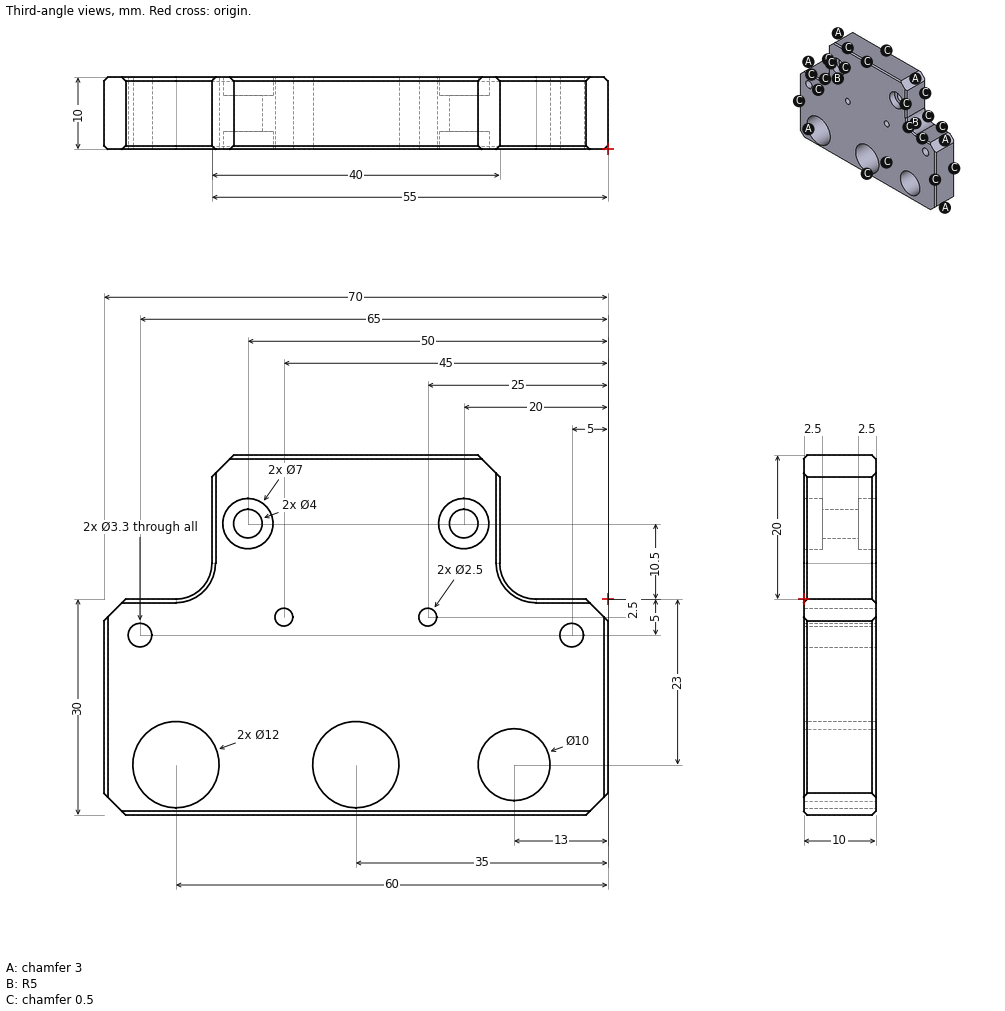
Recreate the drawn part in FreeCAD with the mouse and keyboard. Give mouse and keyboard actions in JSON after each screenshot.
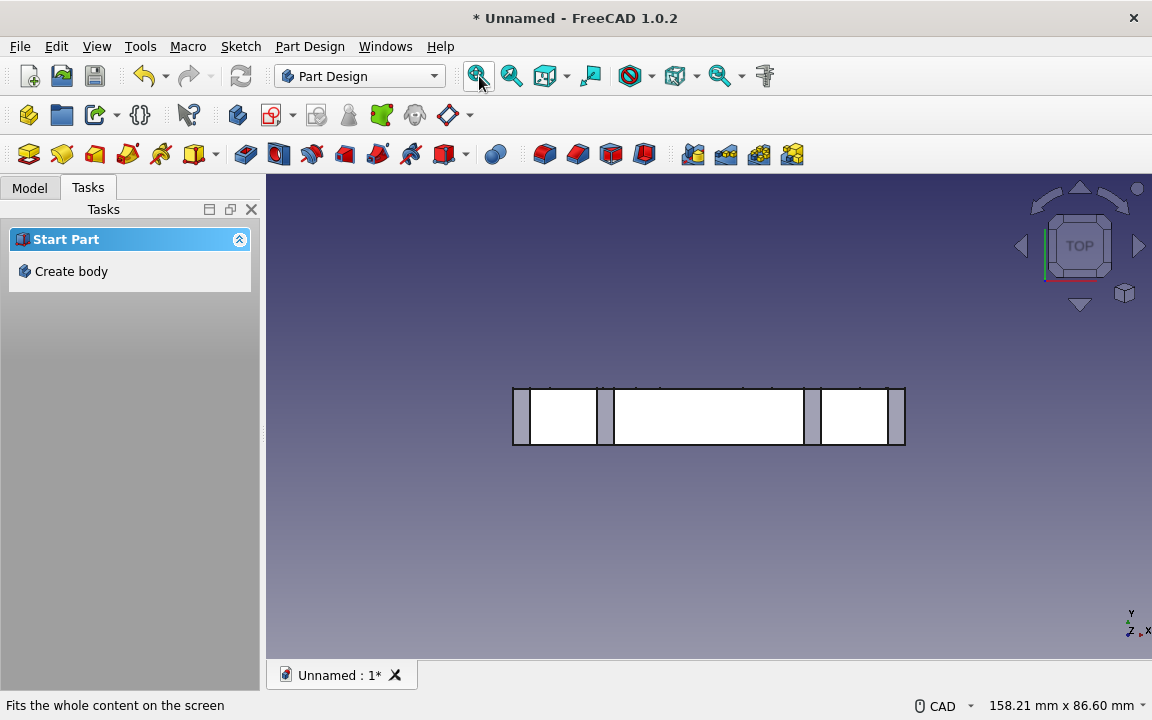
{"action": "left_click", "coordinate": [479, 76]}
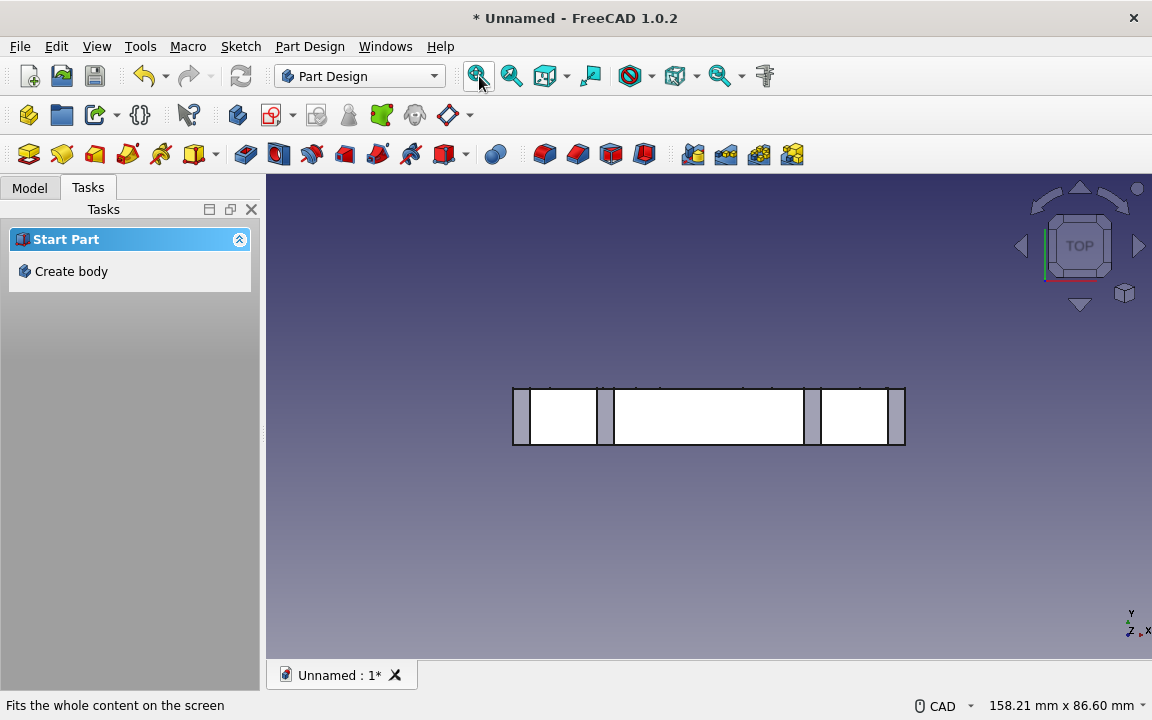
{"action": "key", "text": "1"}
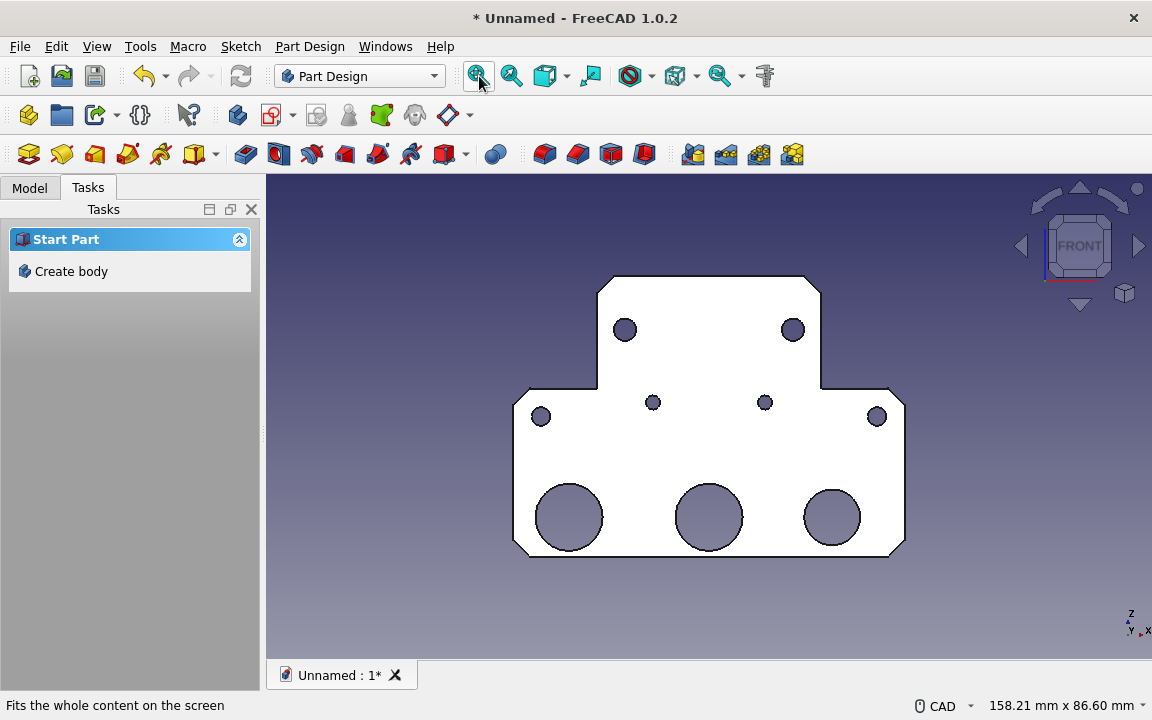
{"action": "key", "text": "3"}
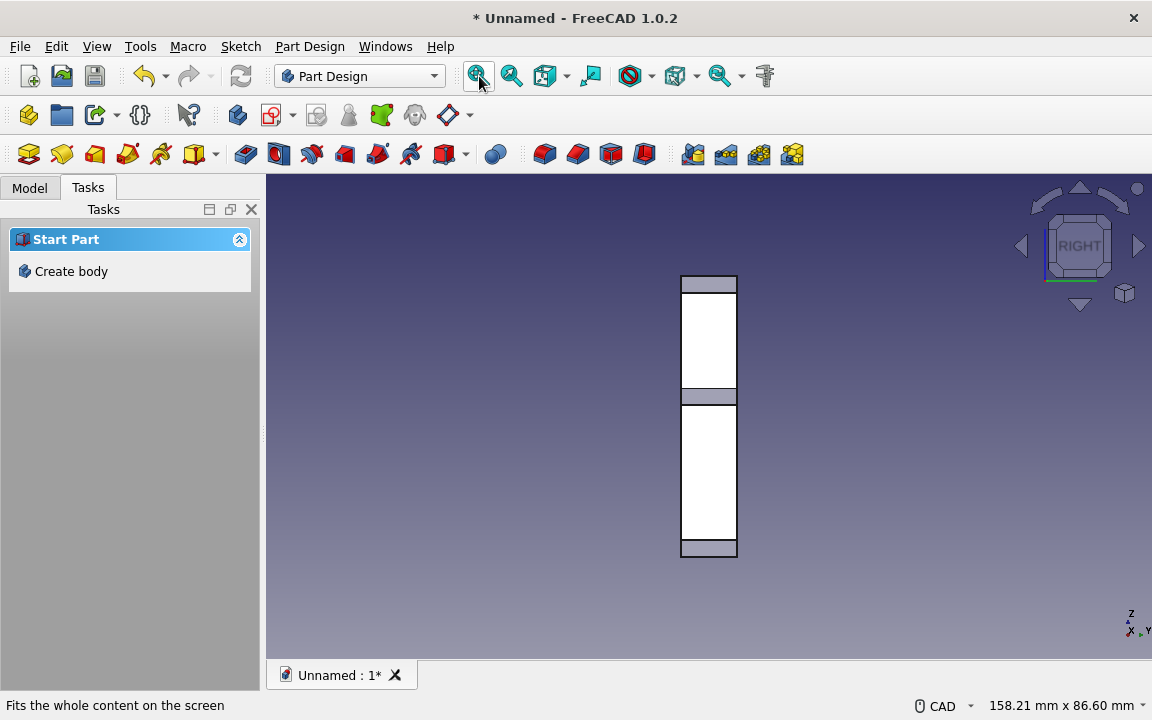
{"action": "key", "text": "5"}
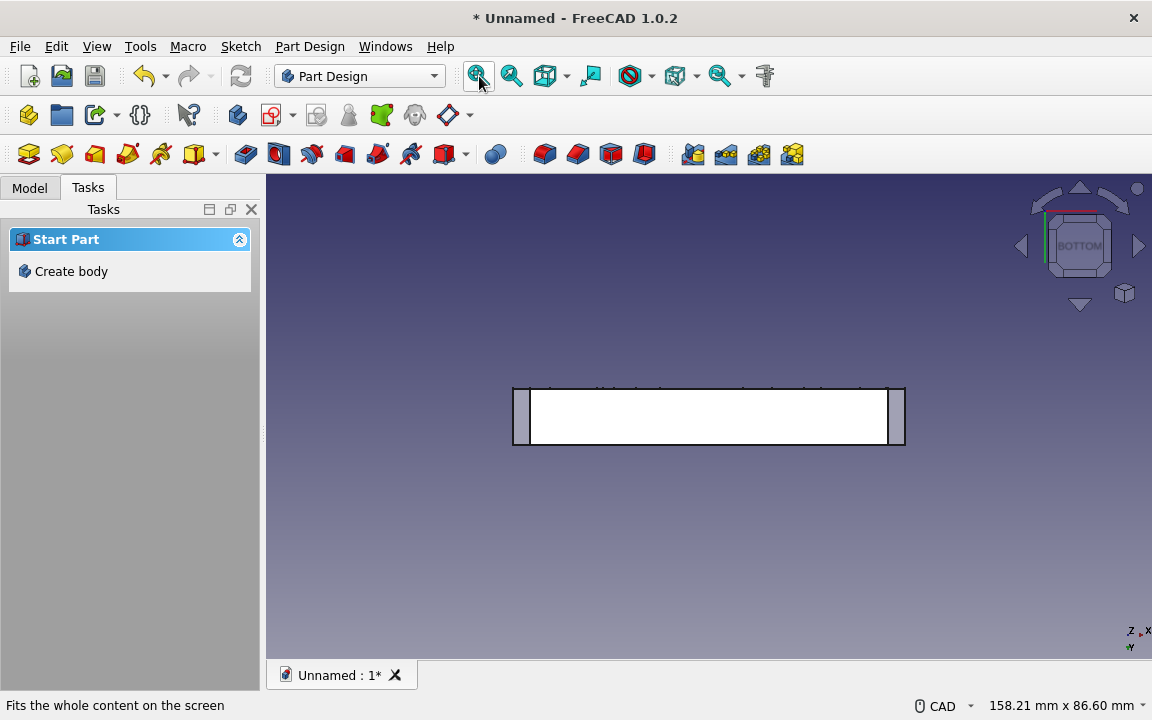
{"action": "left_click", "coordinate": [479, 76]}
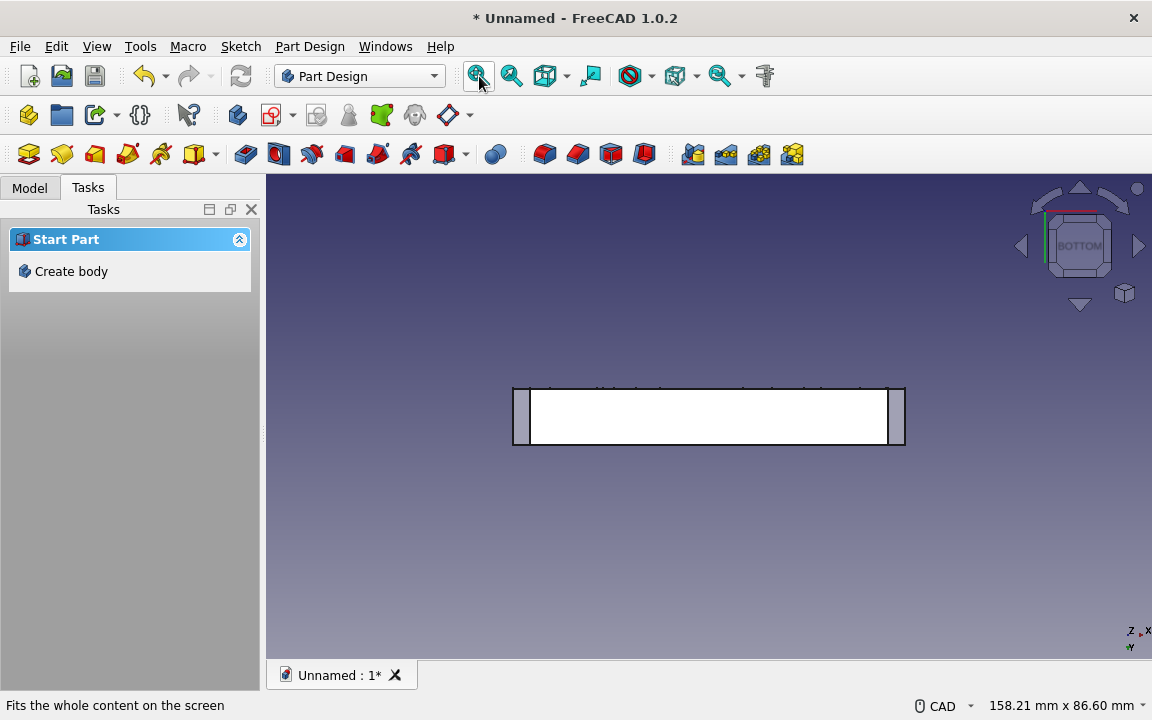
{"action": "key", "text": "4"}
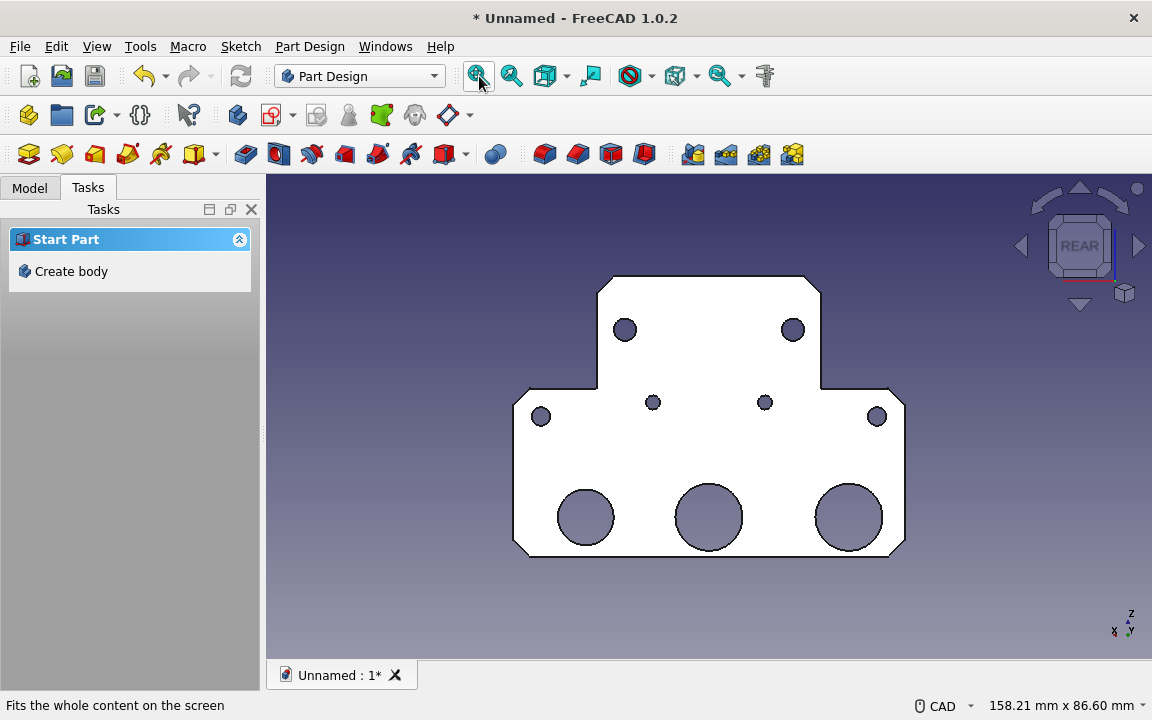
{"action": "key", "text": "6"}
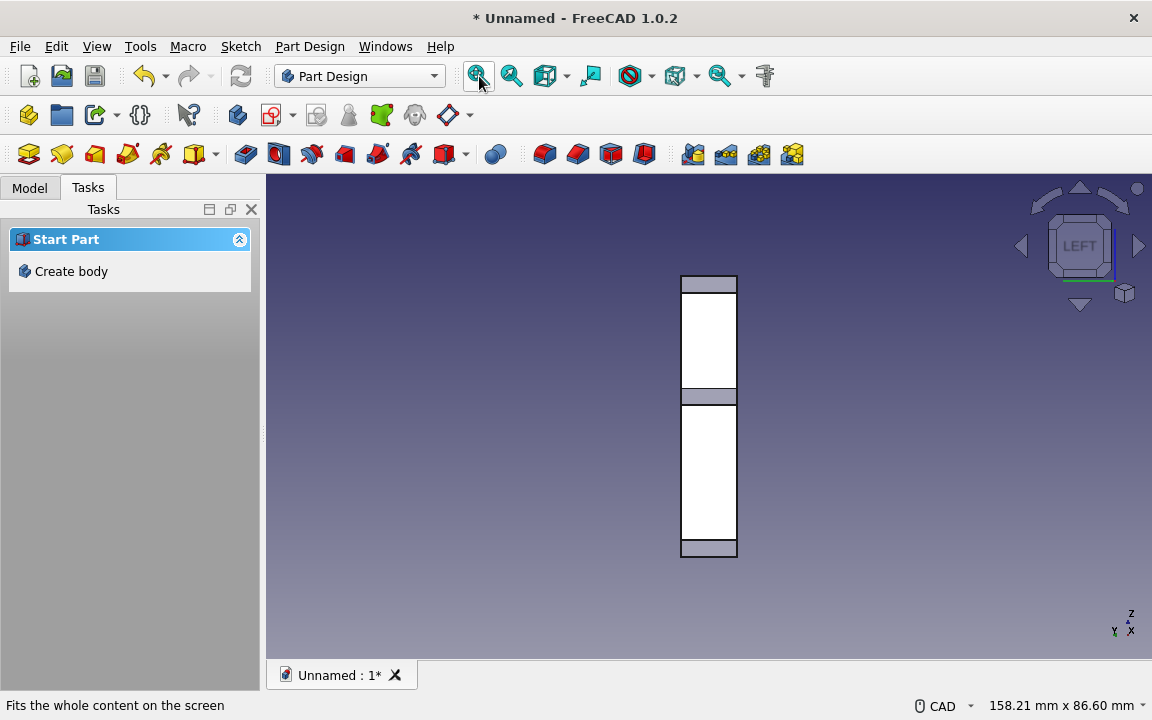
{"action": "key", "text": "v 3"}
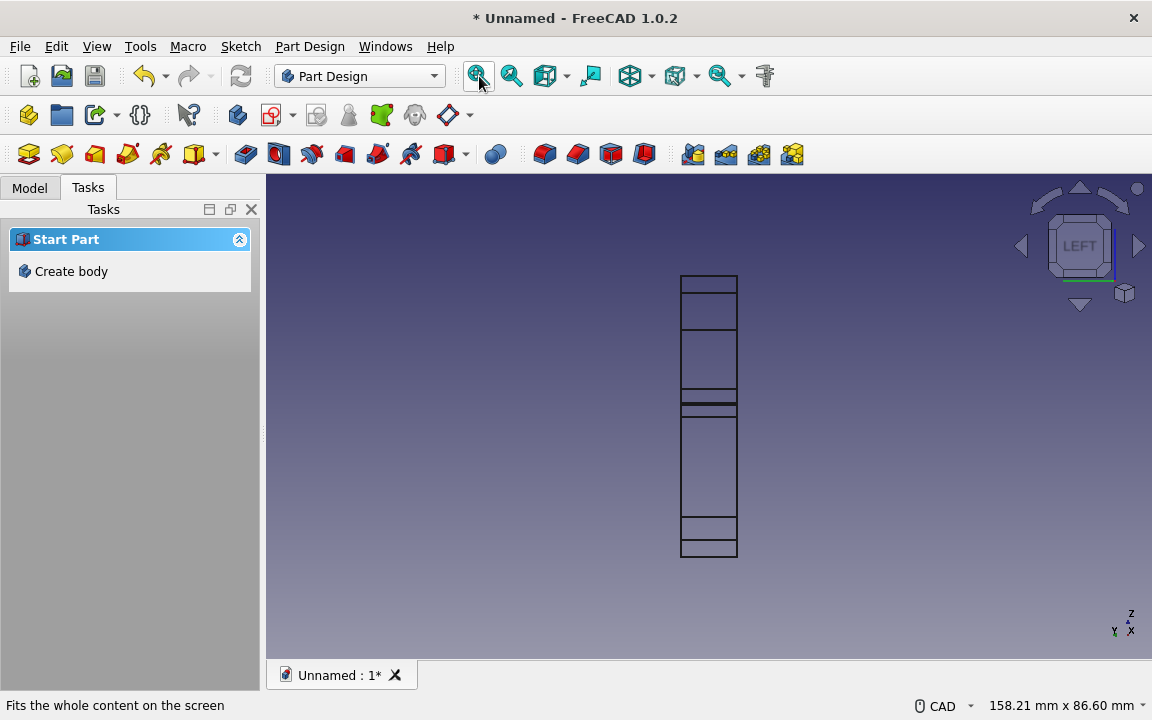
{"action": "key", "text": "0"}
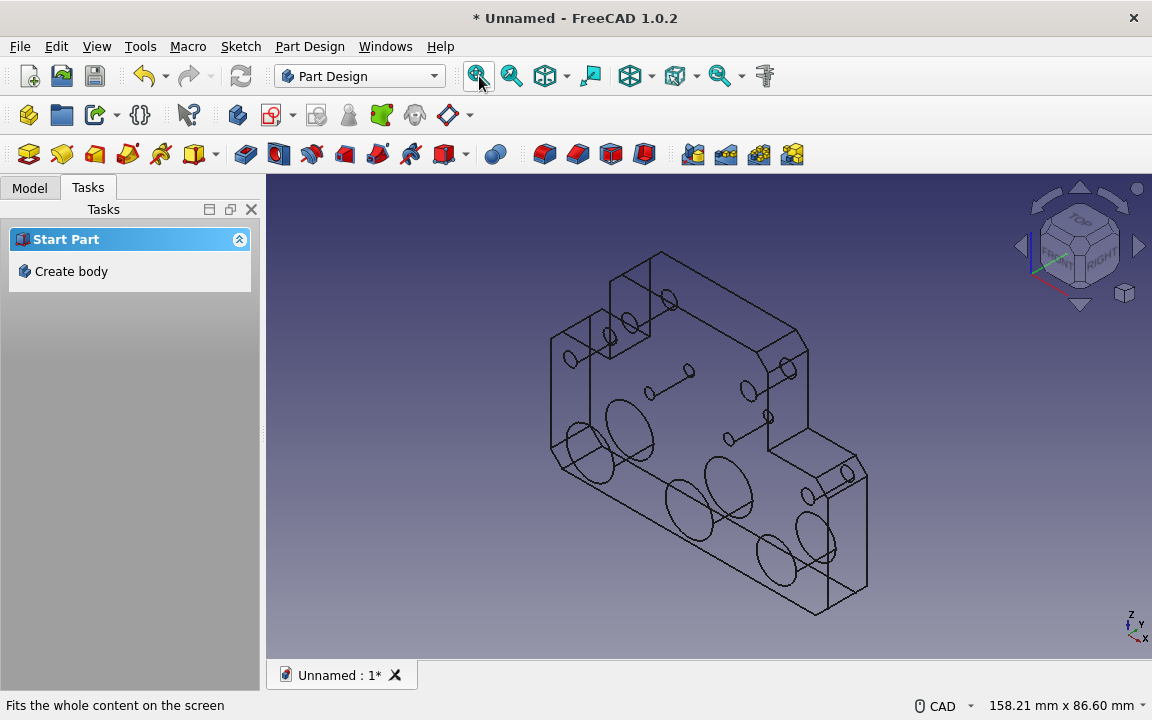
{"action": "left_click", "coordinate": [788, 438]}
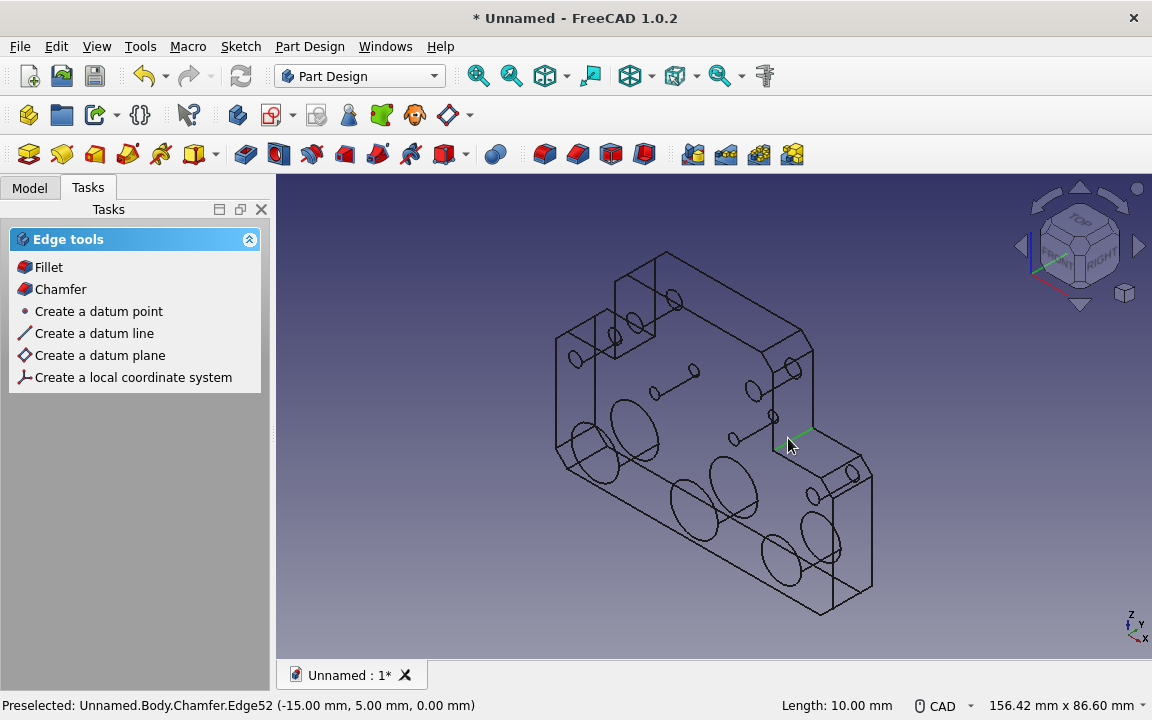
{"action": "left_click", "coordinate": [635, 347], "text": "ctrl"}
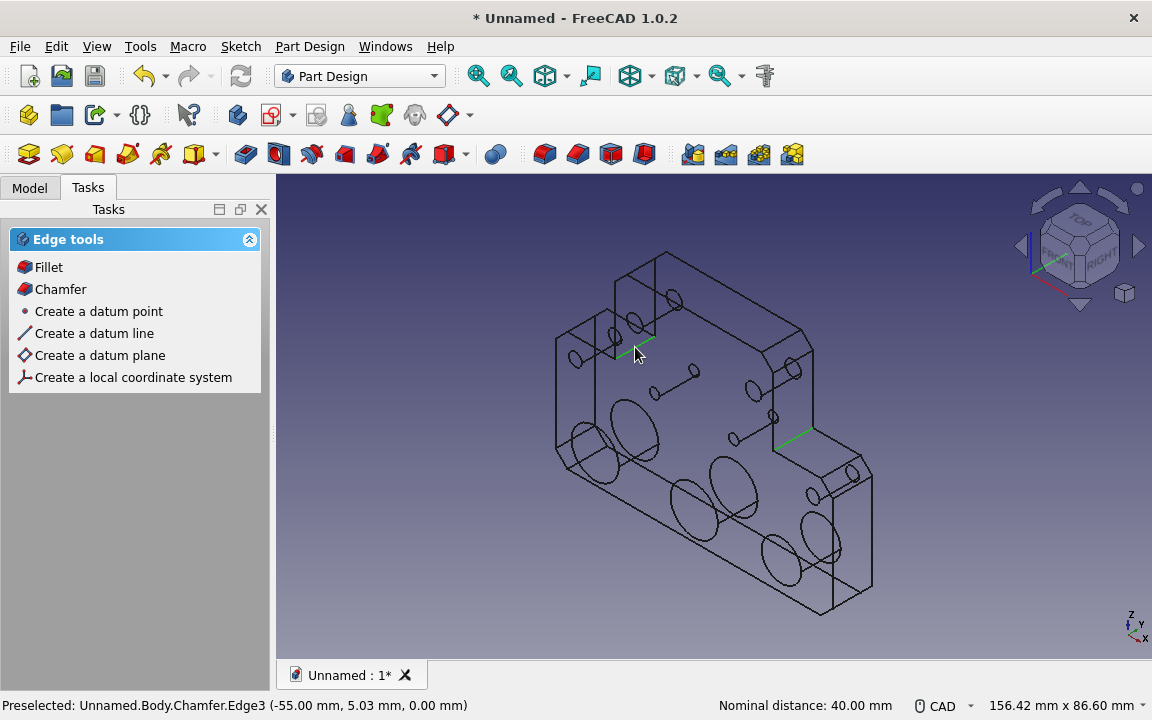
{"action": "key", "text": "v 1"}